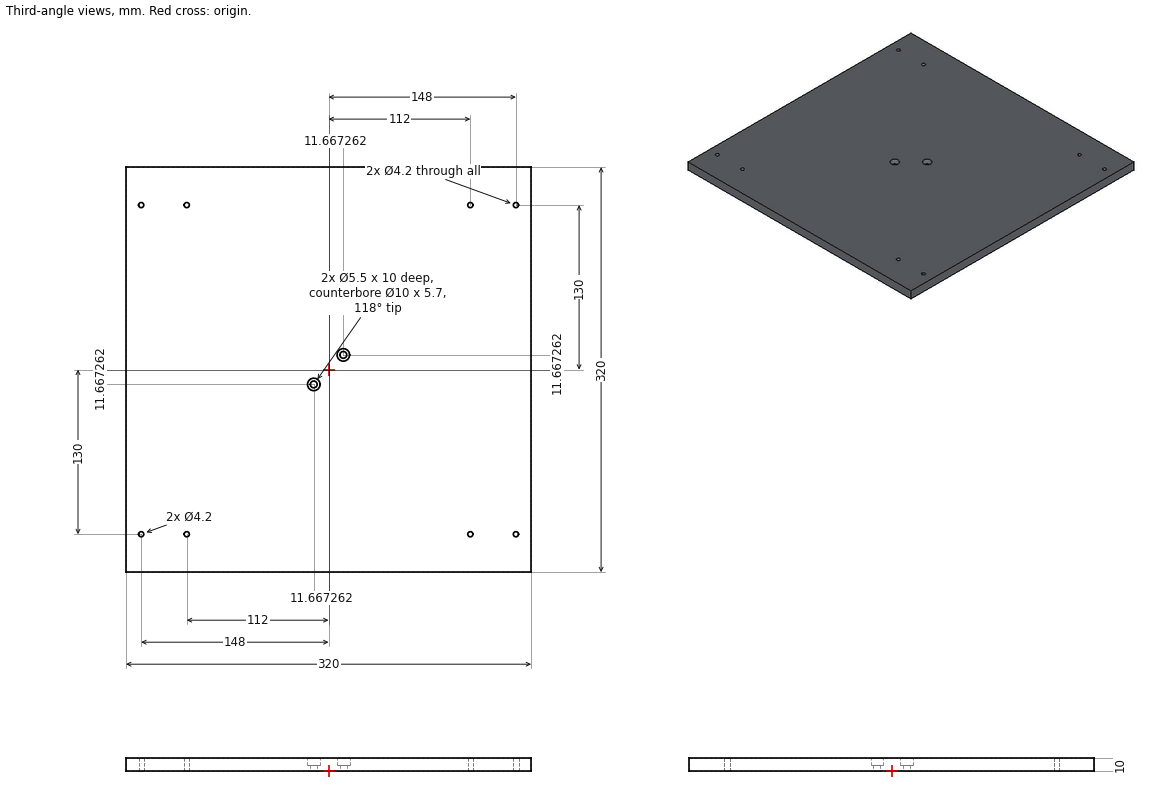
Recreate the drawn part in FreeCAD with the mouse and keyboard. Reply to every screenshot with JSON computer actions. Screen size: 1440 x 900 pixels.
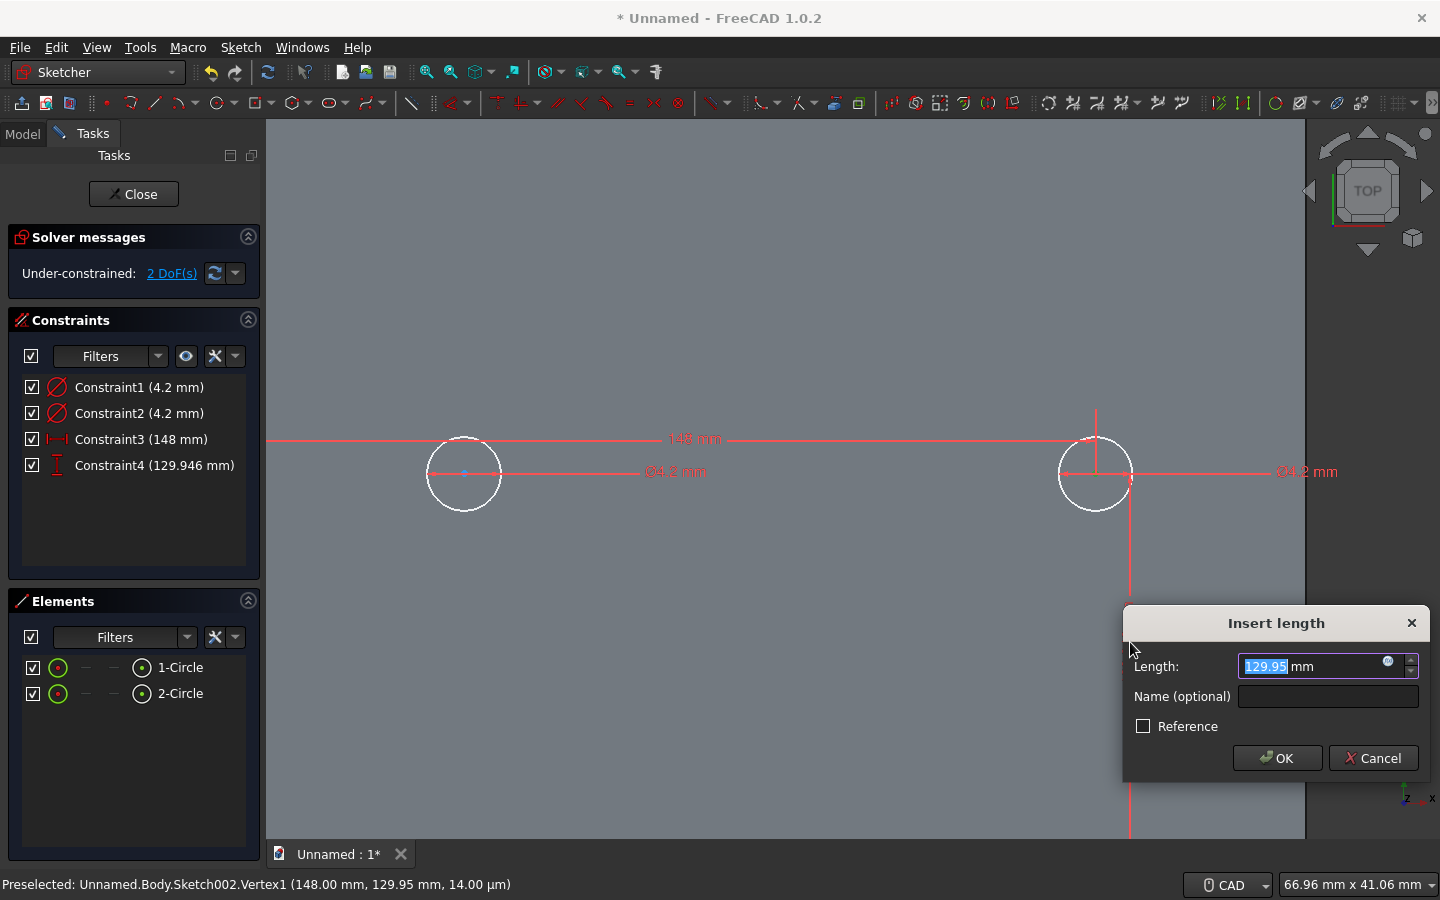
{"action": "type", "text": "130"}
{"action": "key", "text": "Return"}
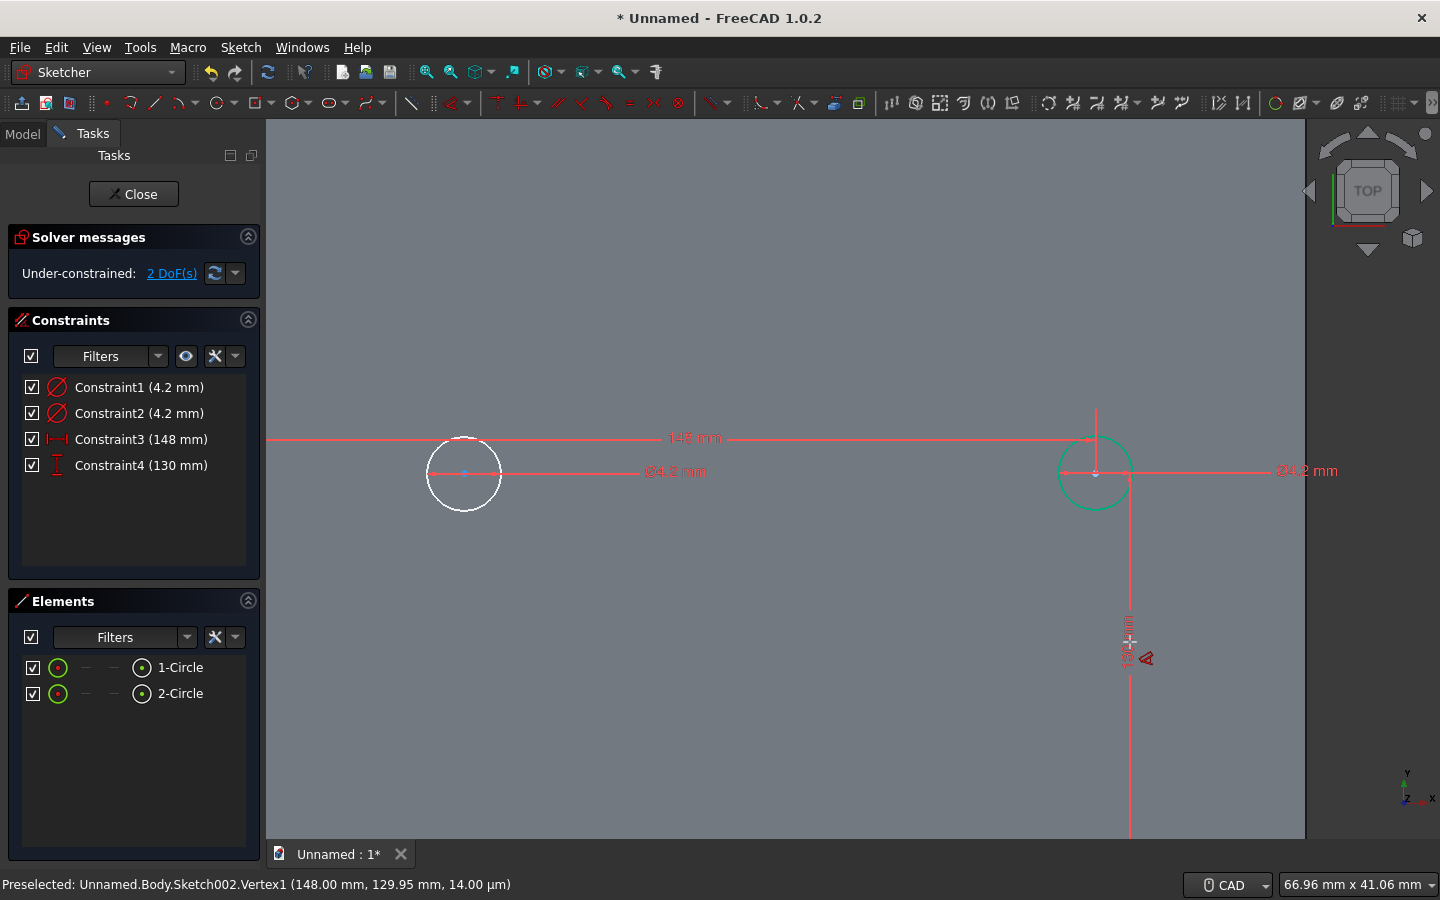
{"action": "left_click", "coordinate": [464, 474]}
{"action": "left_click", "coordinate": [379, 440]}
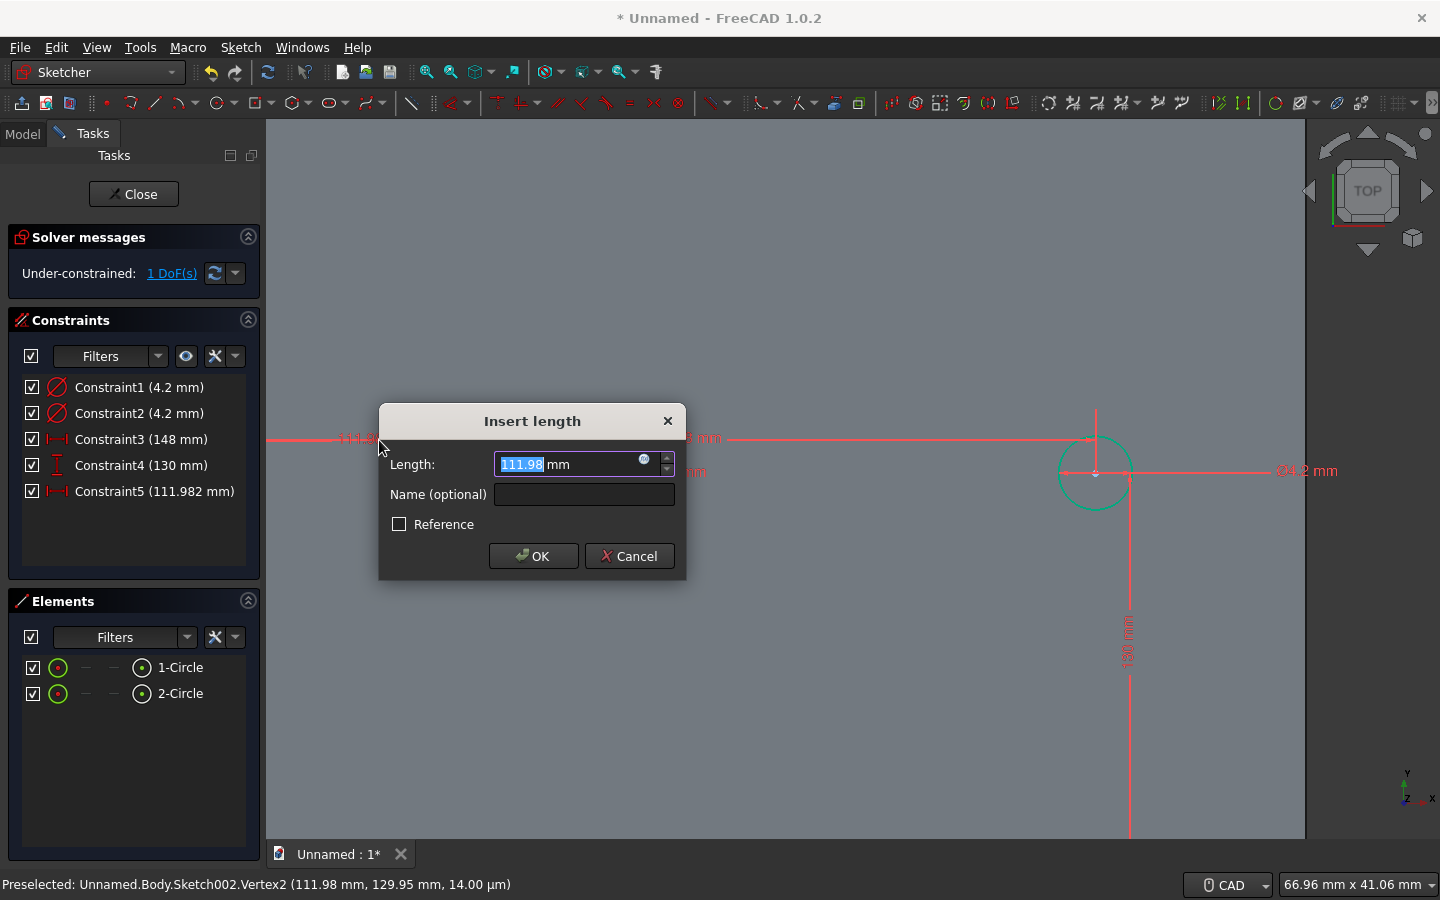
{"action": "type", "text": "112"}
{"action": "key", "text": "Return"}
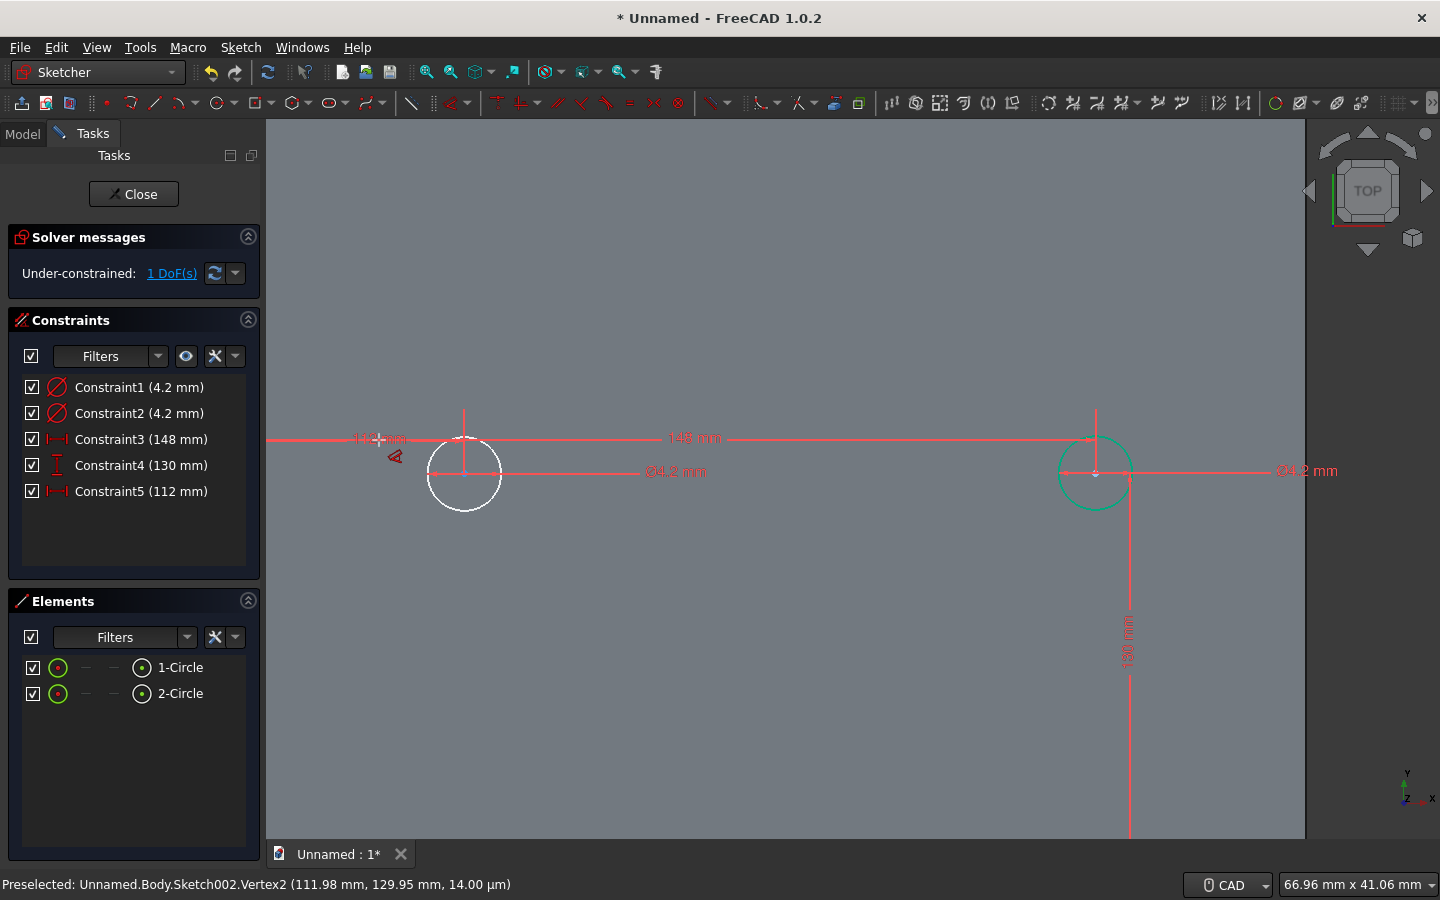
{"action": "left_click", "coordinate": [464, 474]}
{"action": "left_click", "coordinate": [498, 642]}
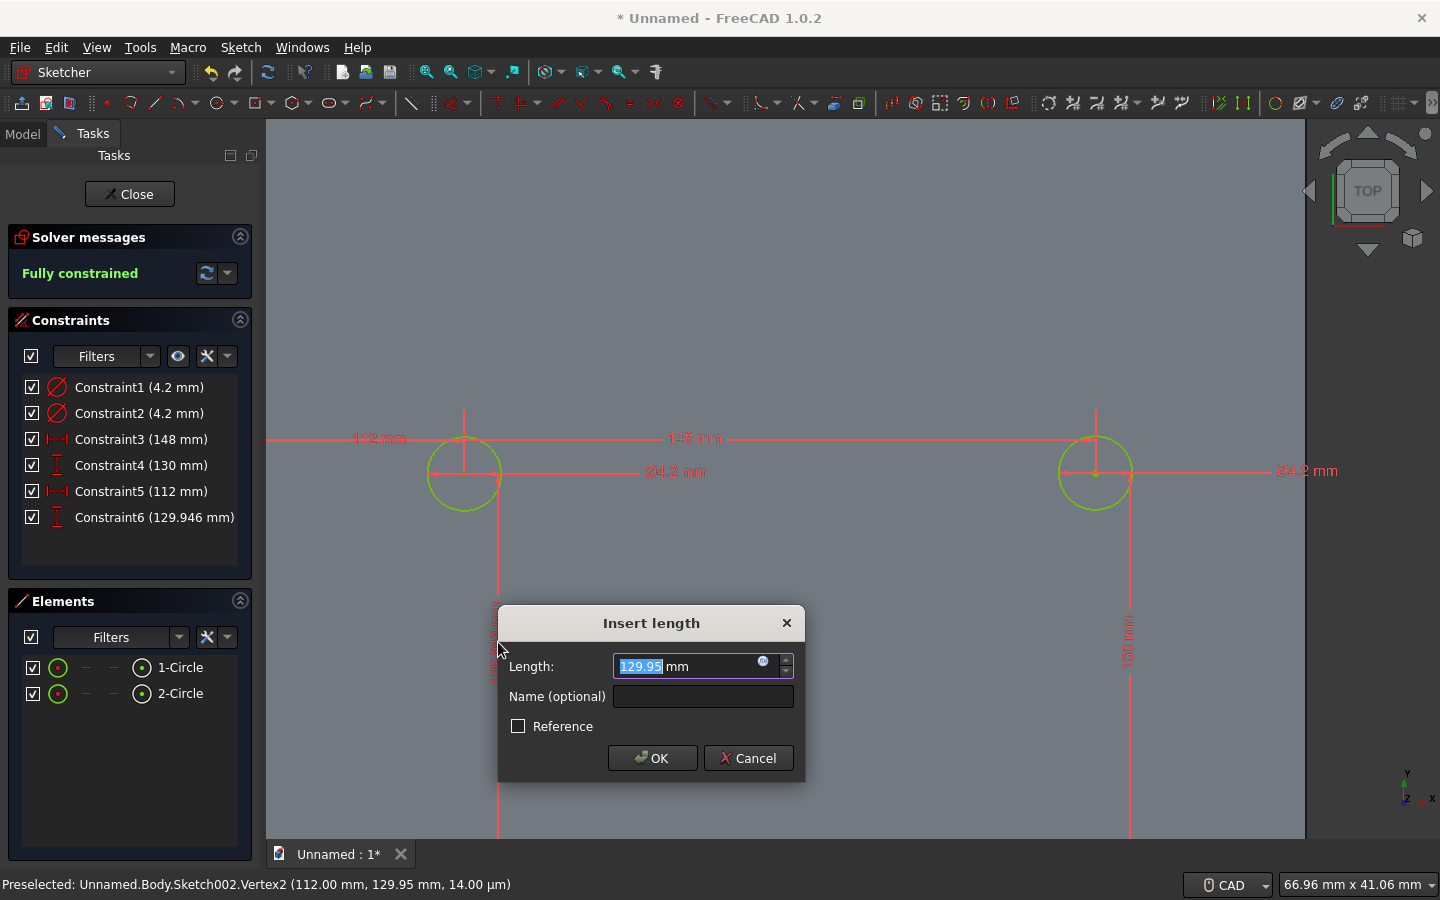
{"action": "type", "text": "130"}
{"action": "key", "text": "Return"}
{"action": "key", "text": "Escape"}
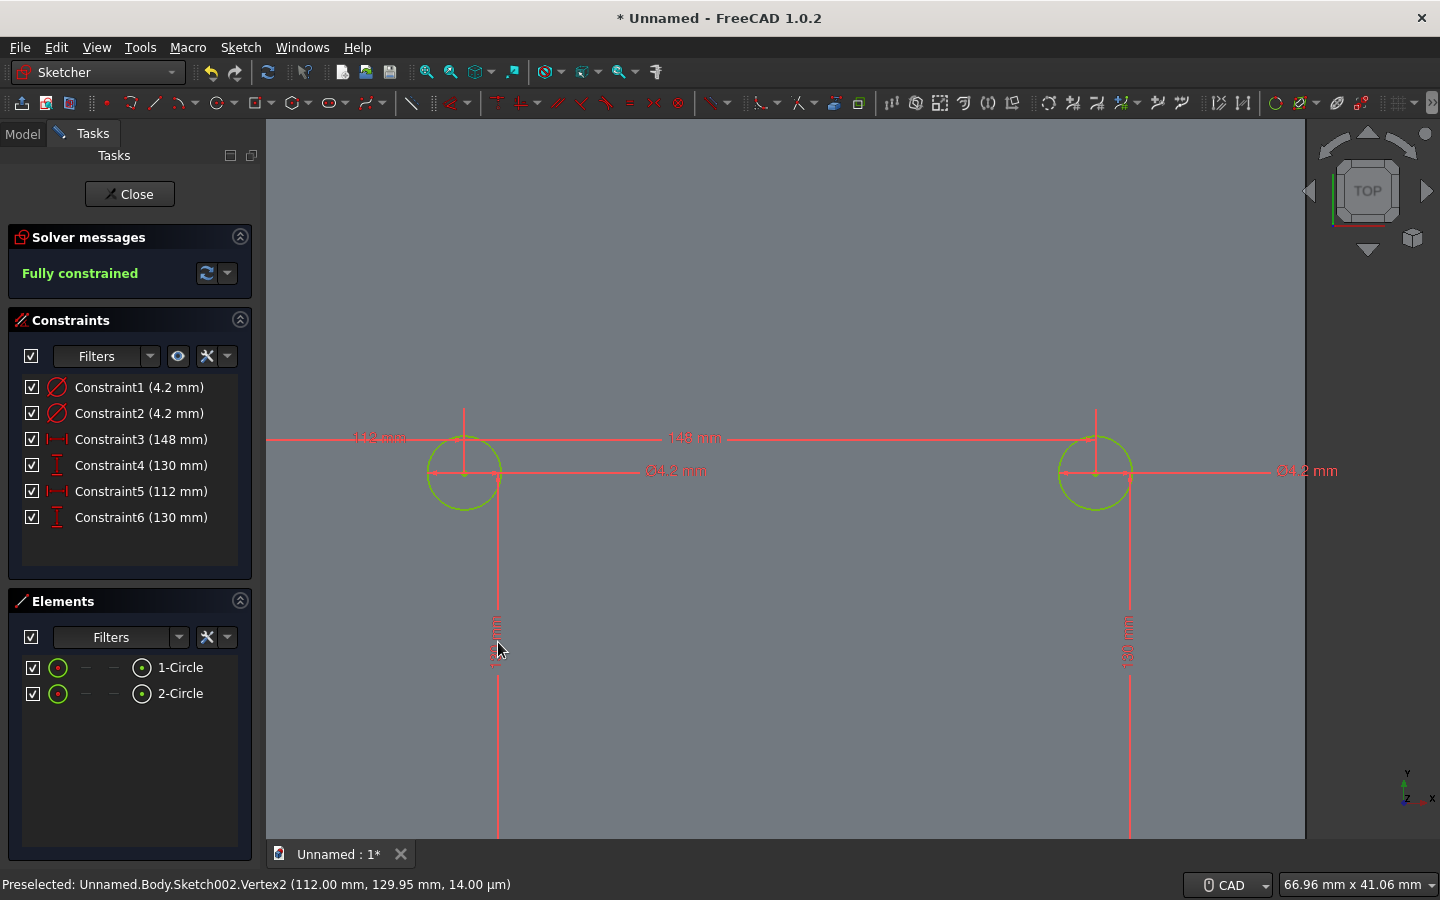
{"action": "left_click", "coordinate": [130, 194]}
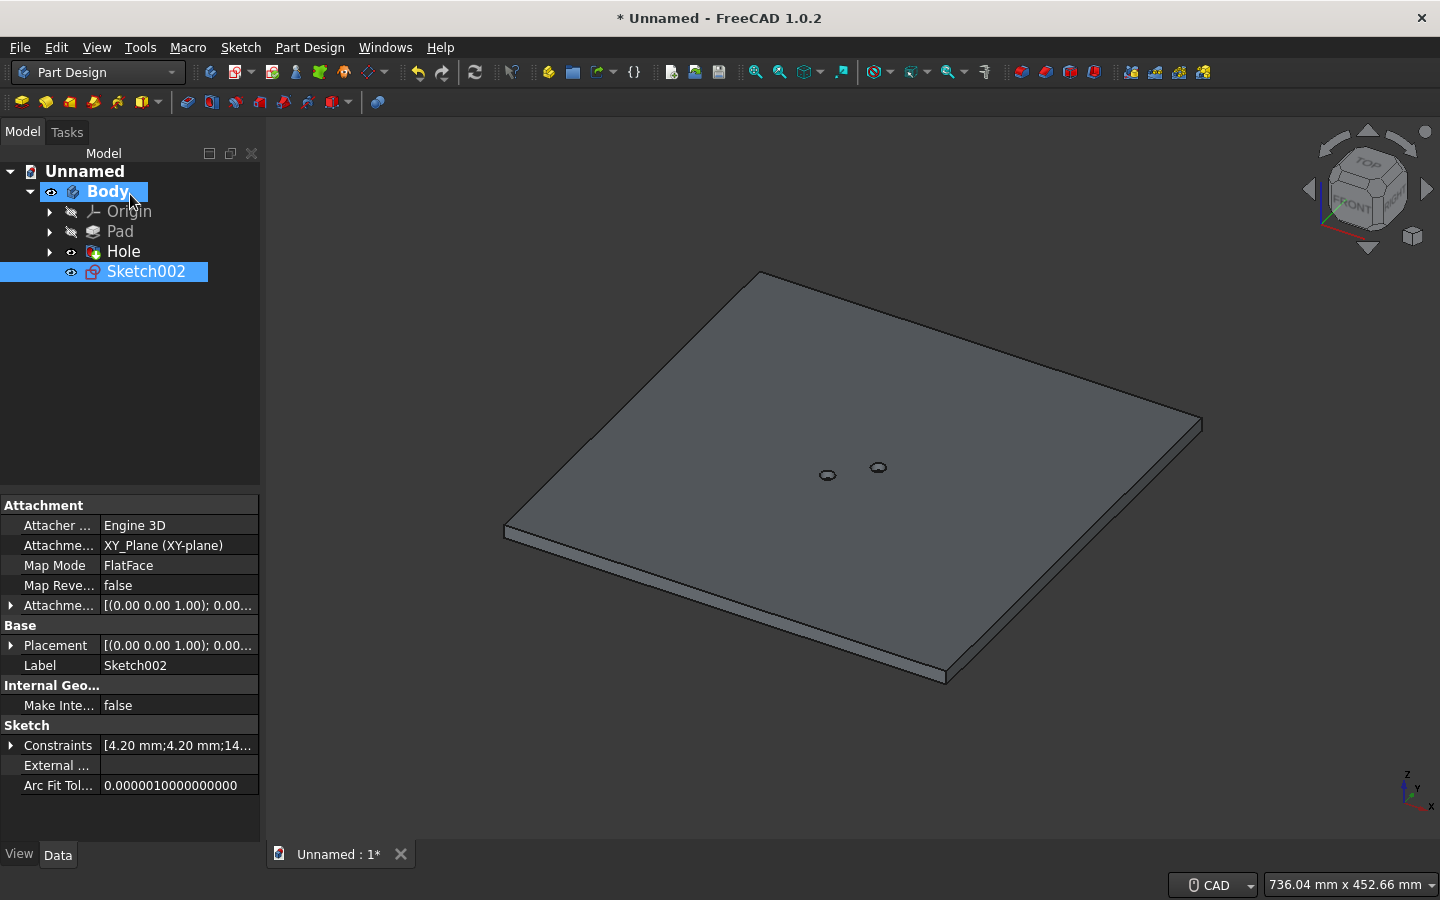
{"action": "left_click", "coordinate": [212, 102]}